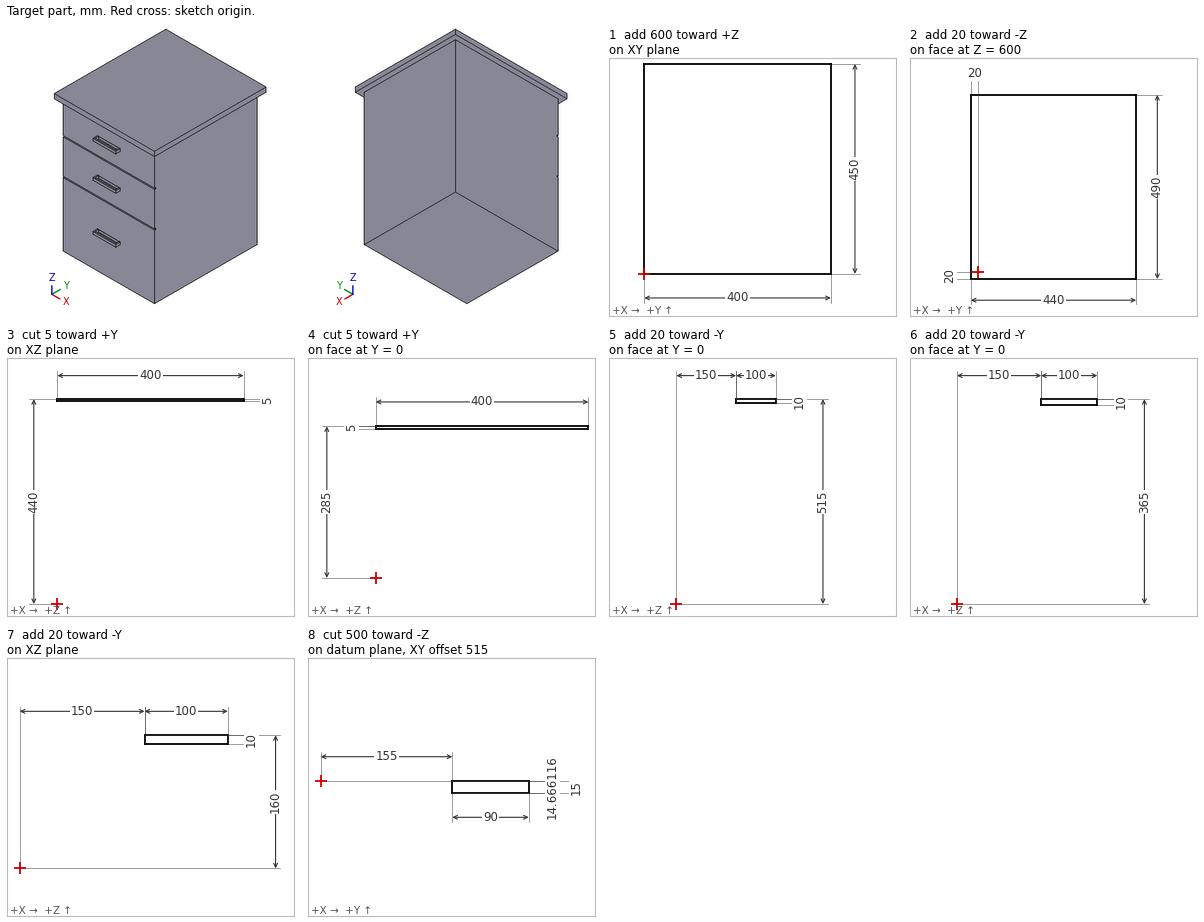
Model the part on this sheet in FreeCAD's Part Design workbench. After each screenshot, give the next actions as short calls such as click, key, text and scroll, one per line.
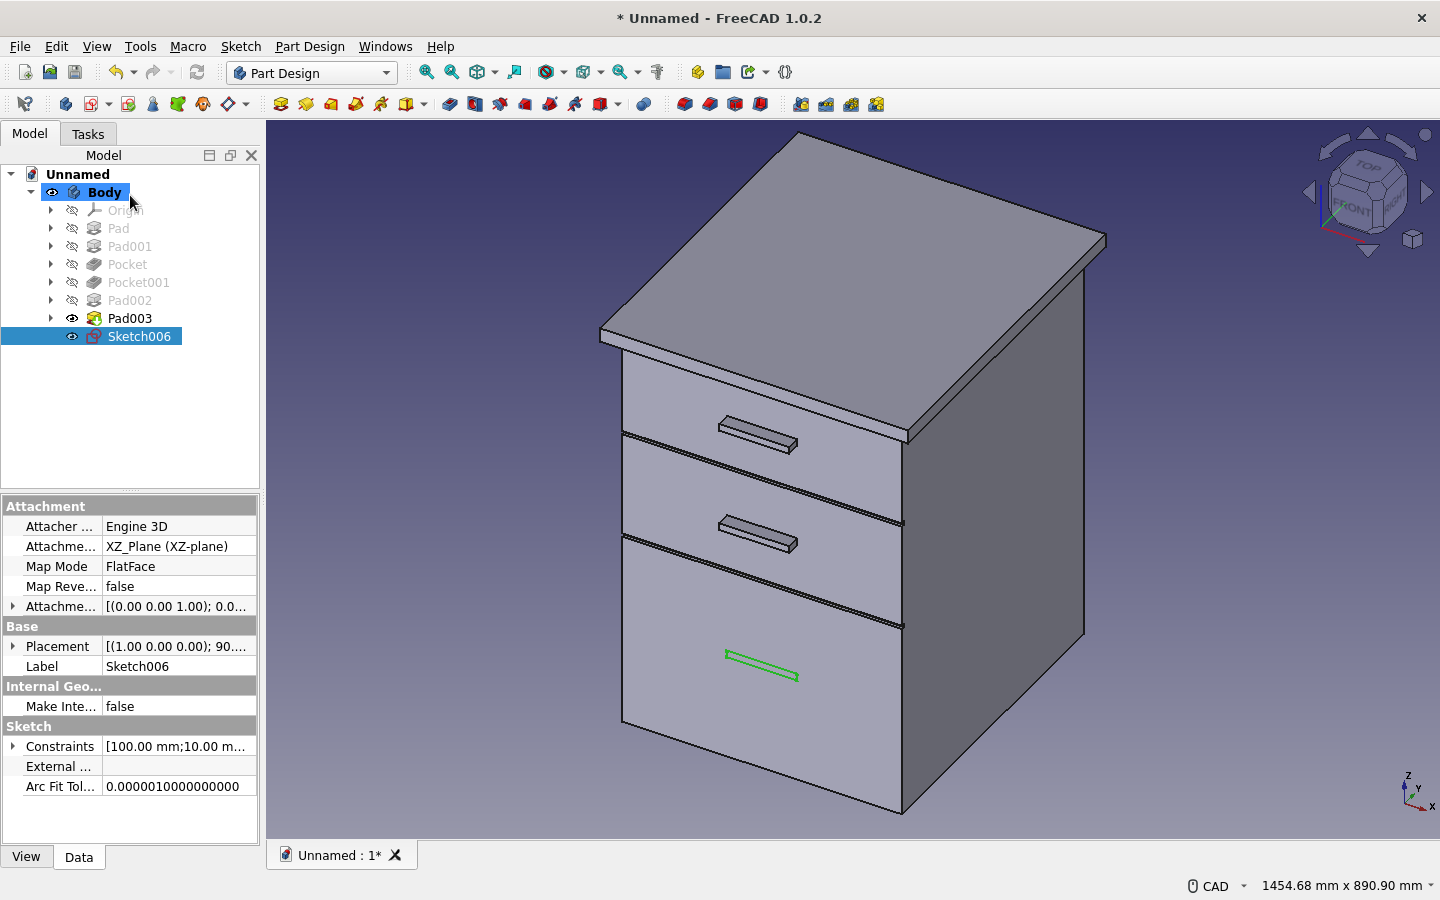
click(281, 104)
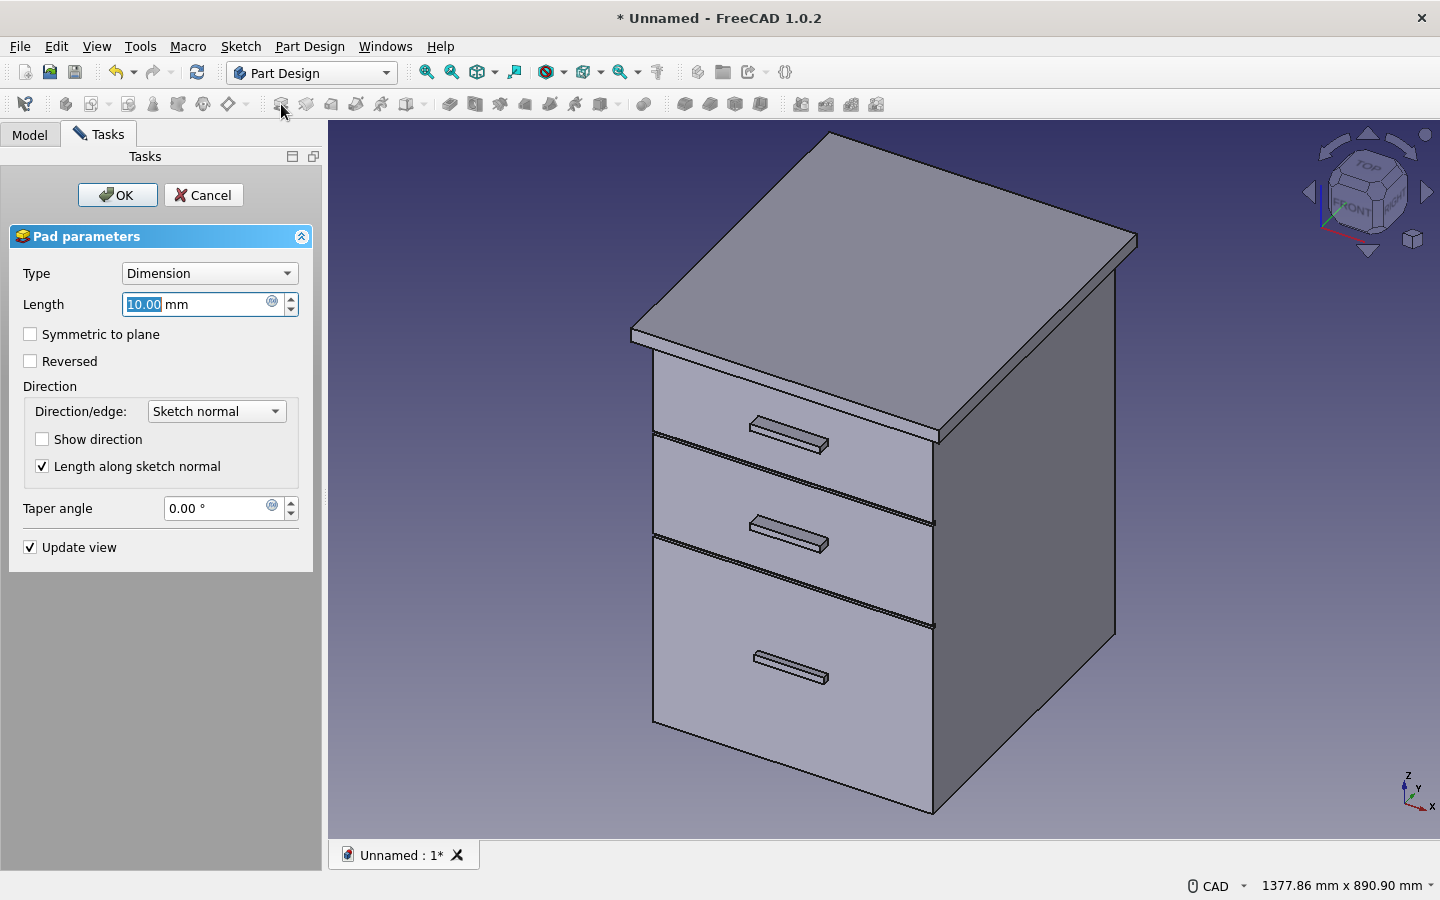
text(20)
key(Tab)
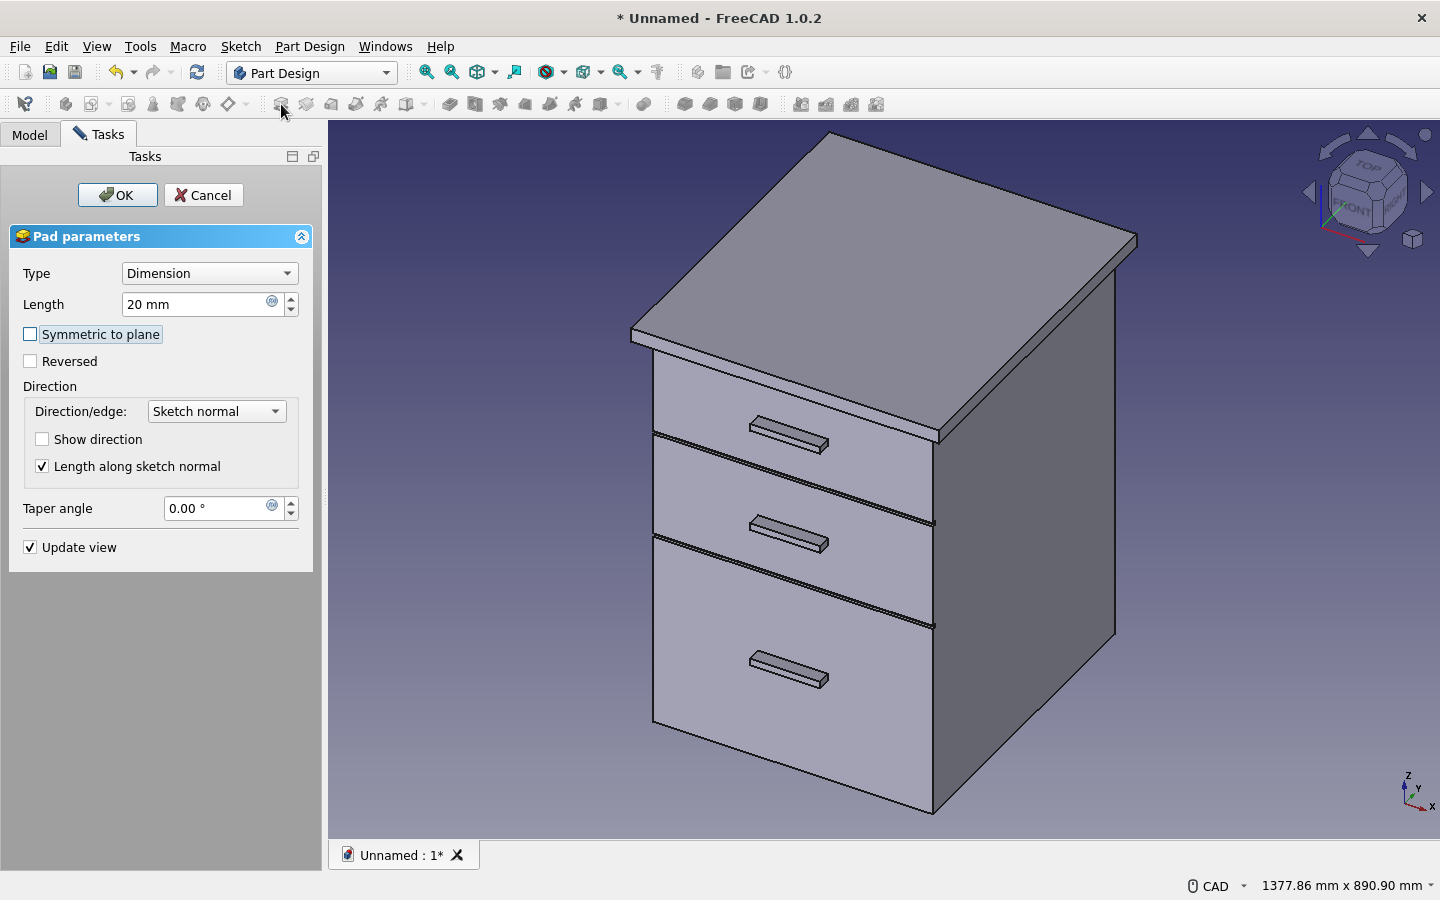
click(118, 195)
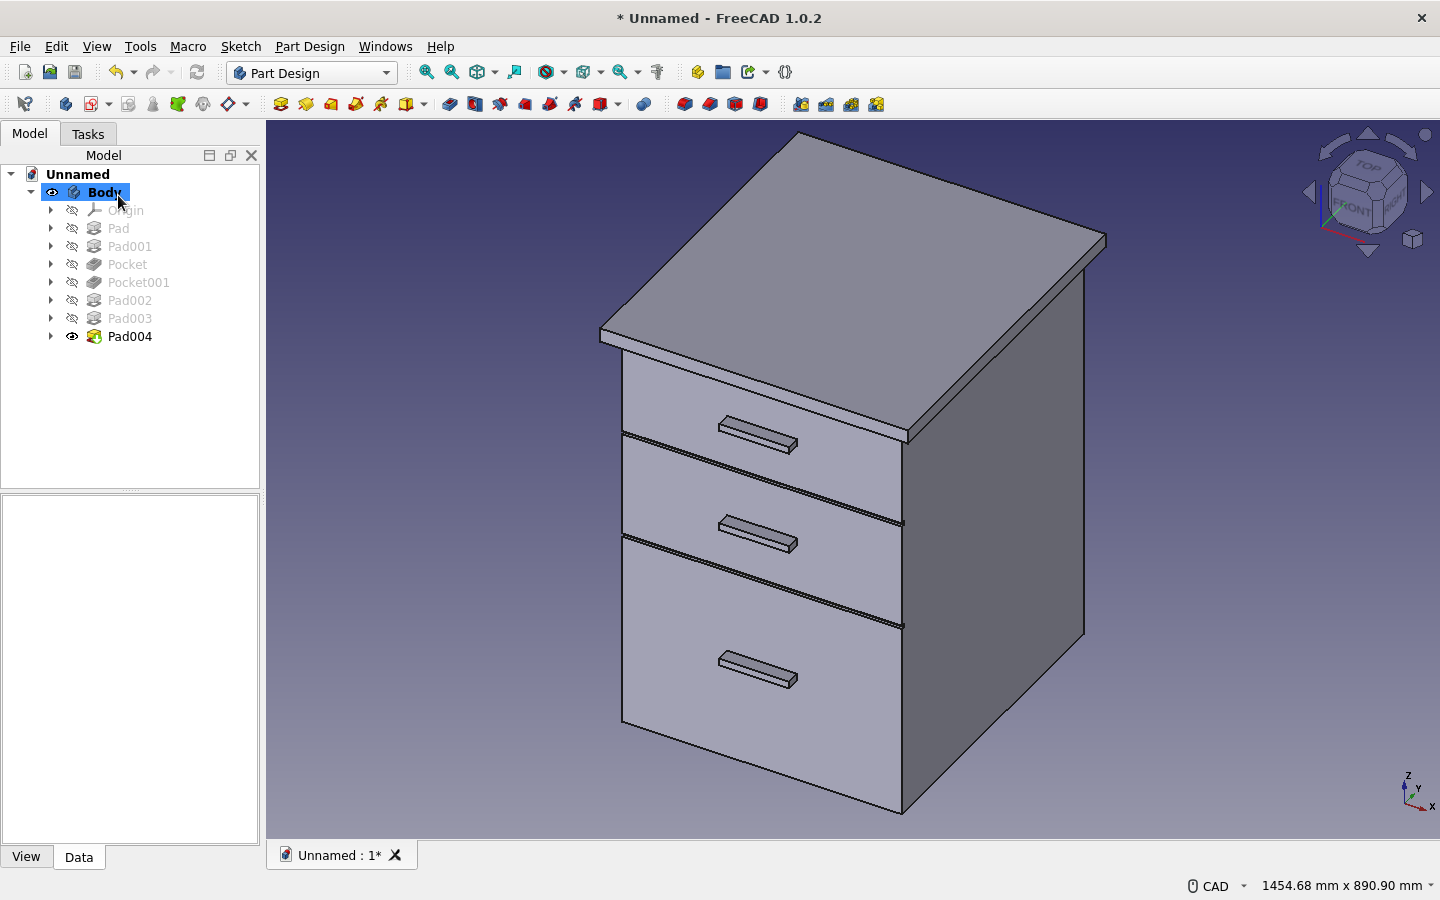
click(51, 210)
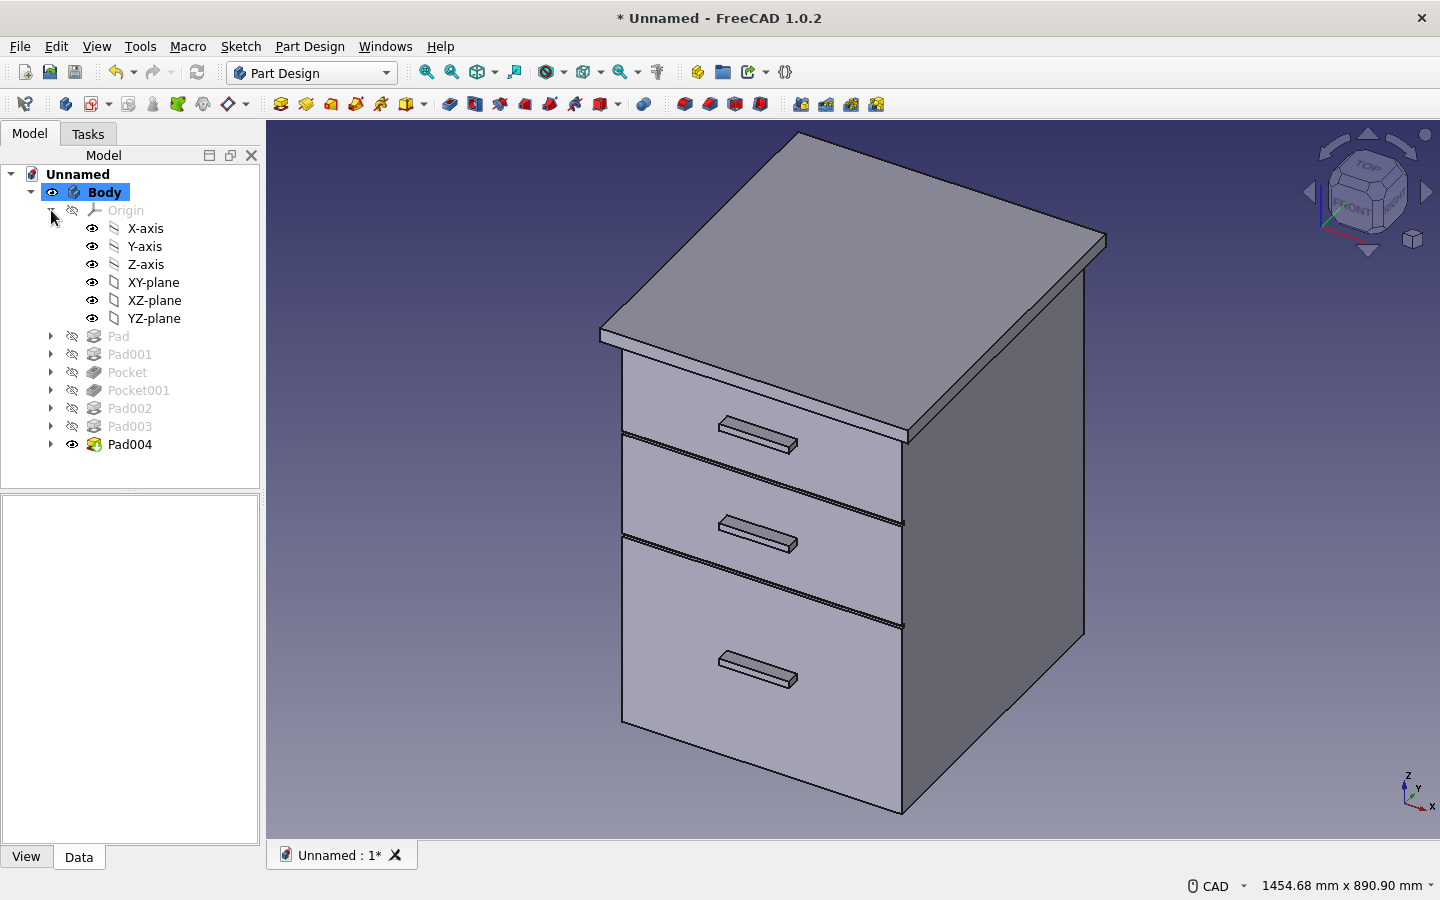
click(137, 282)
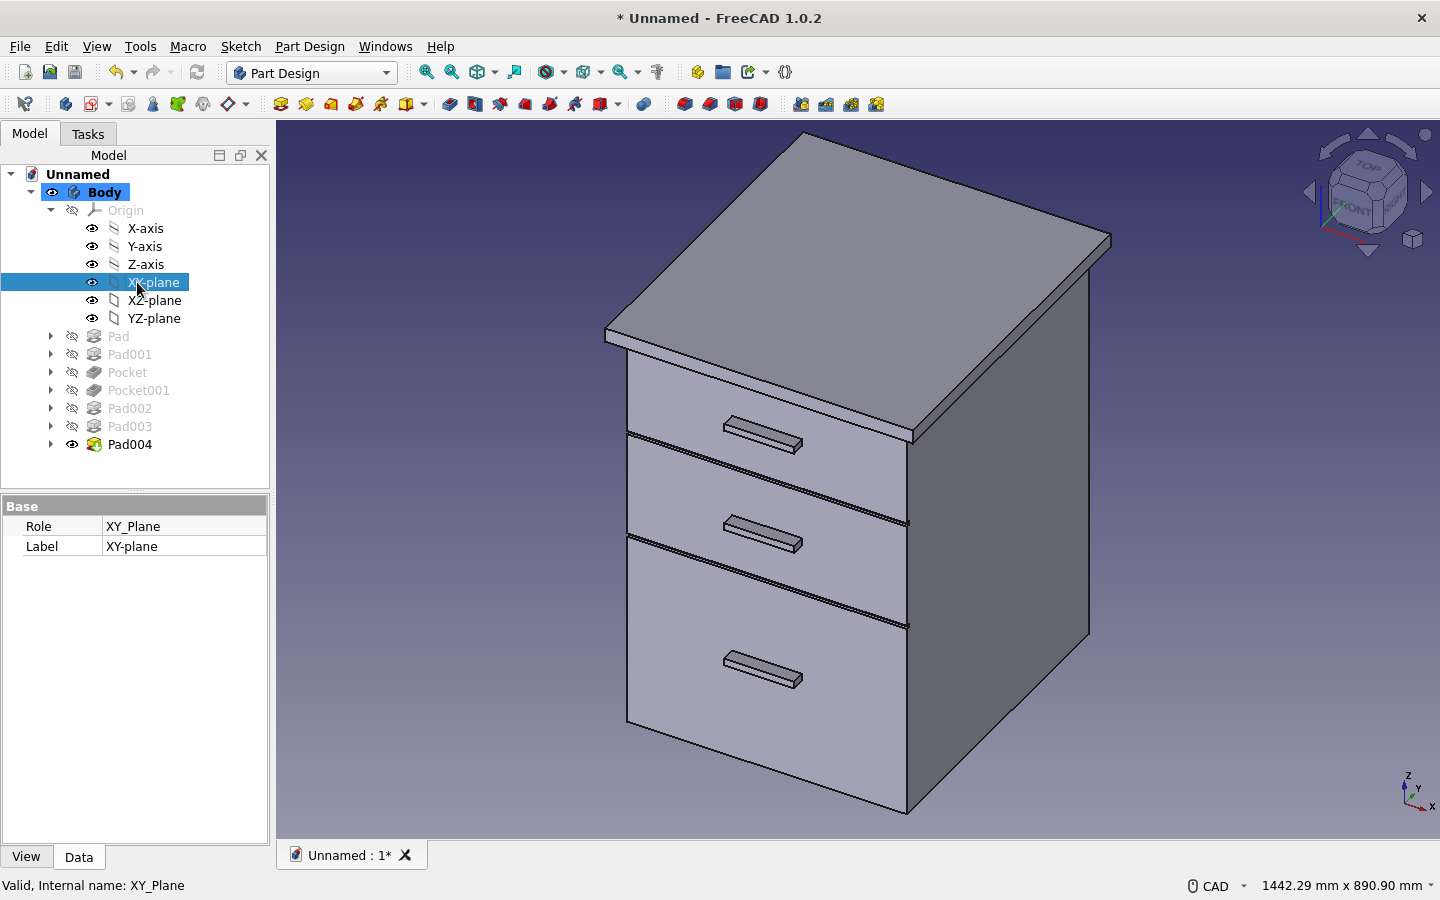
click(228, 104)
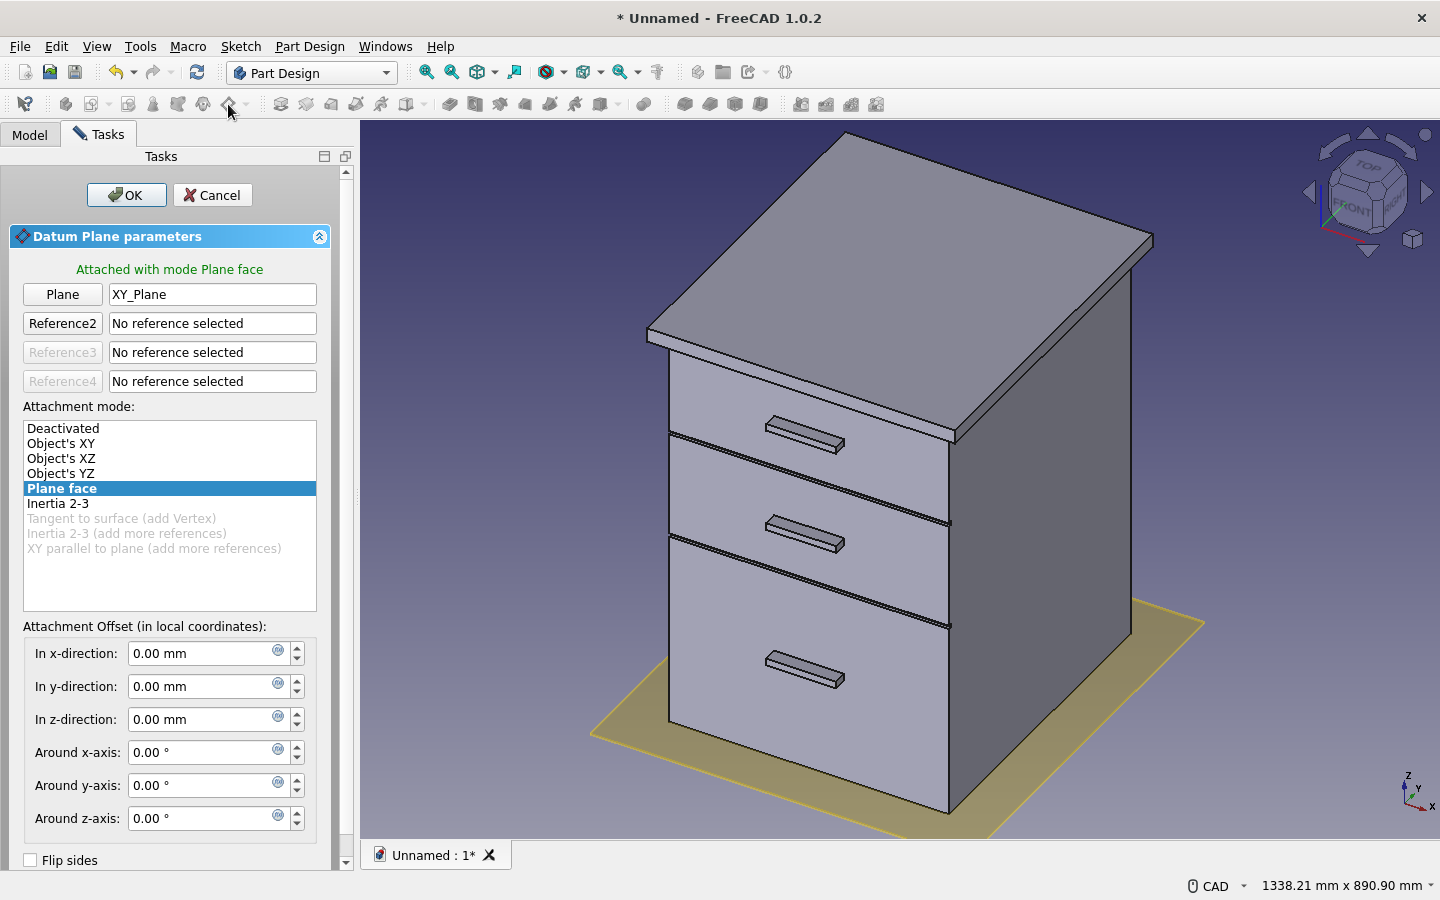
triple_click(210, 720)